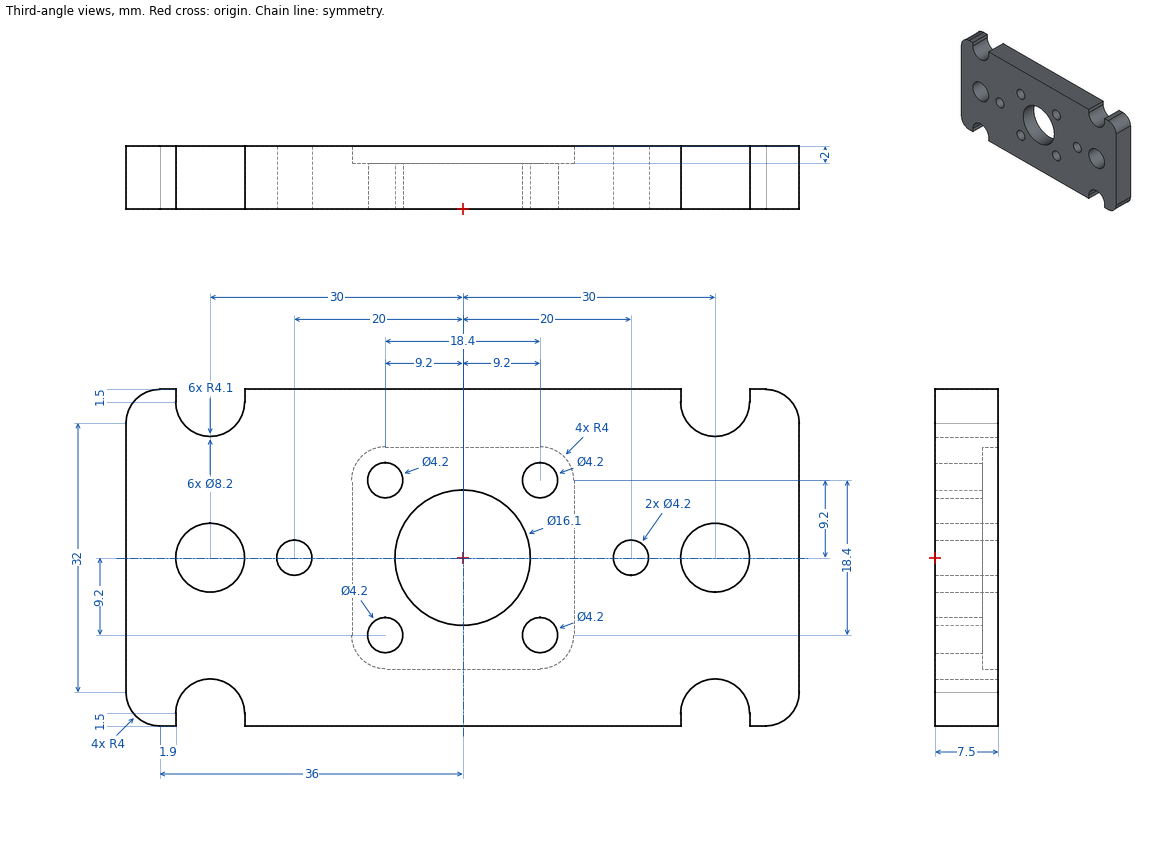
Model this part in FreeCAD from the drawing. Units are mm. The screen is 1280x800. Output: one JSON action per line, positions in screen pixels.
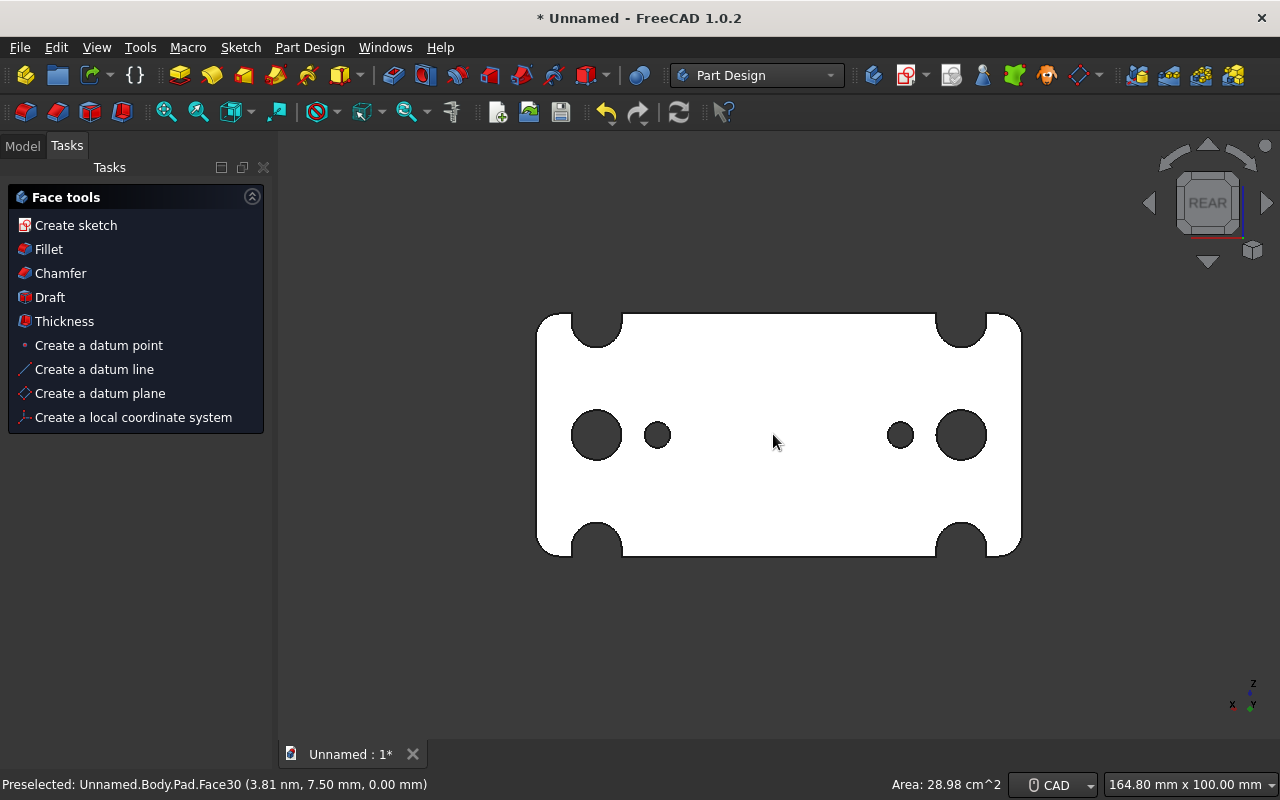
{"action": "left_click", "coordinate": [906, 76]}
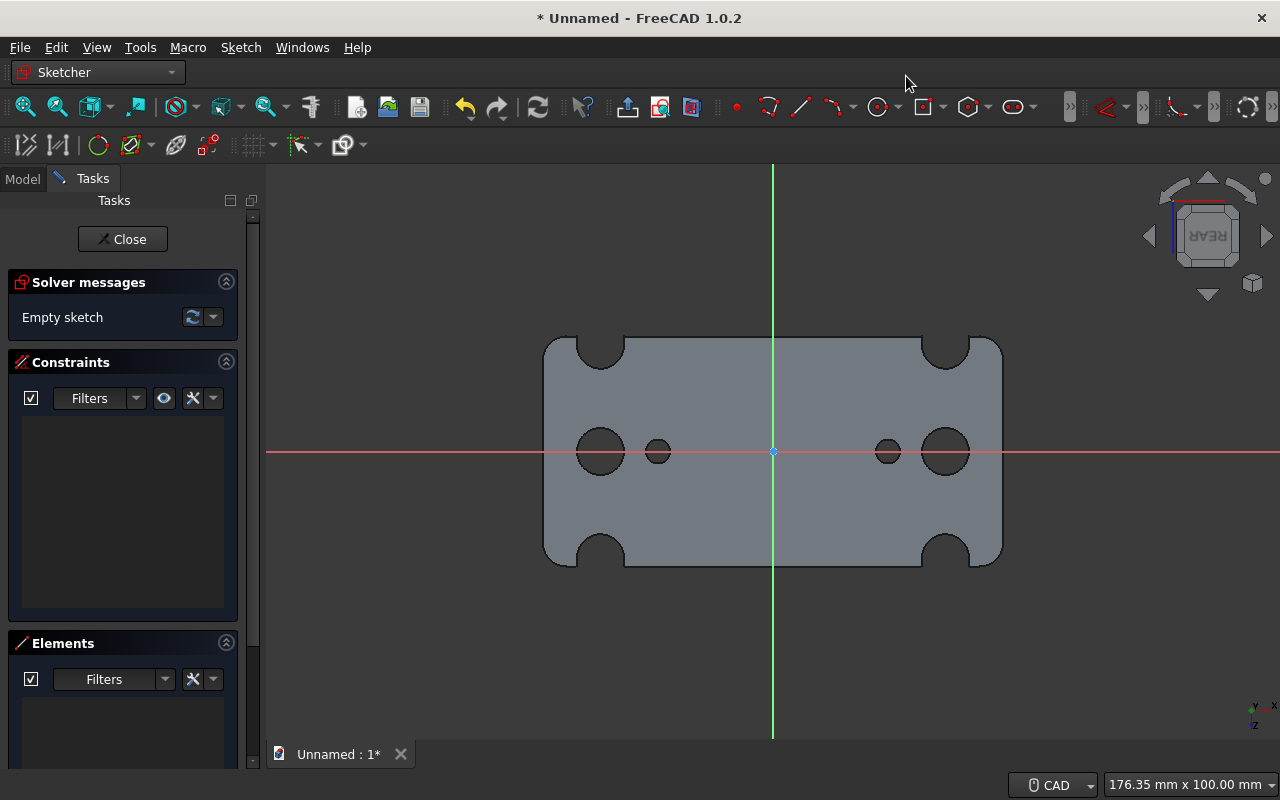
{"action": "scroll", "coordinate": [829, 452], "scroll_direction": "up", "scroll_amount": 4}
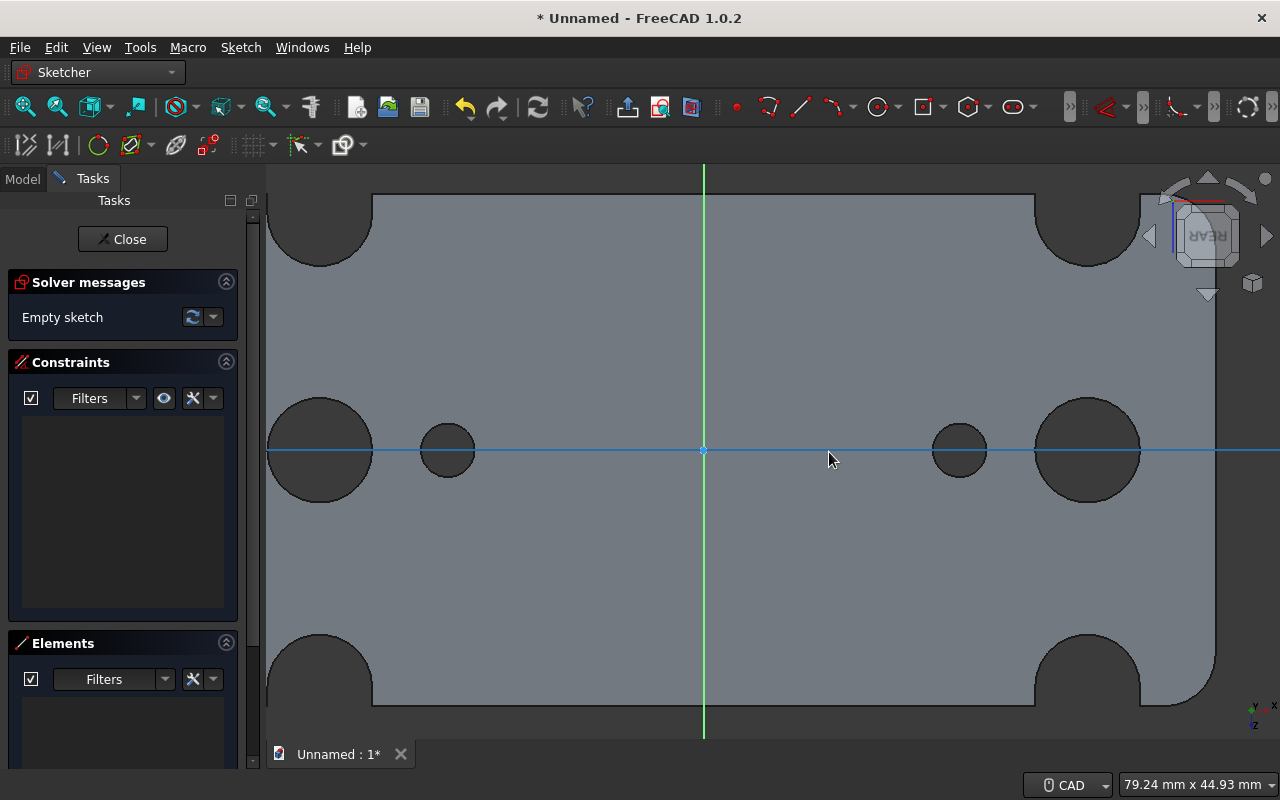
{"action": "left_click", "coordinate": [802, 108]}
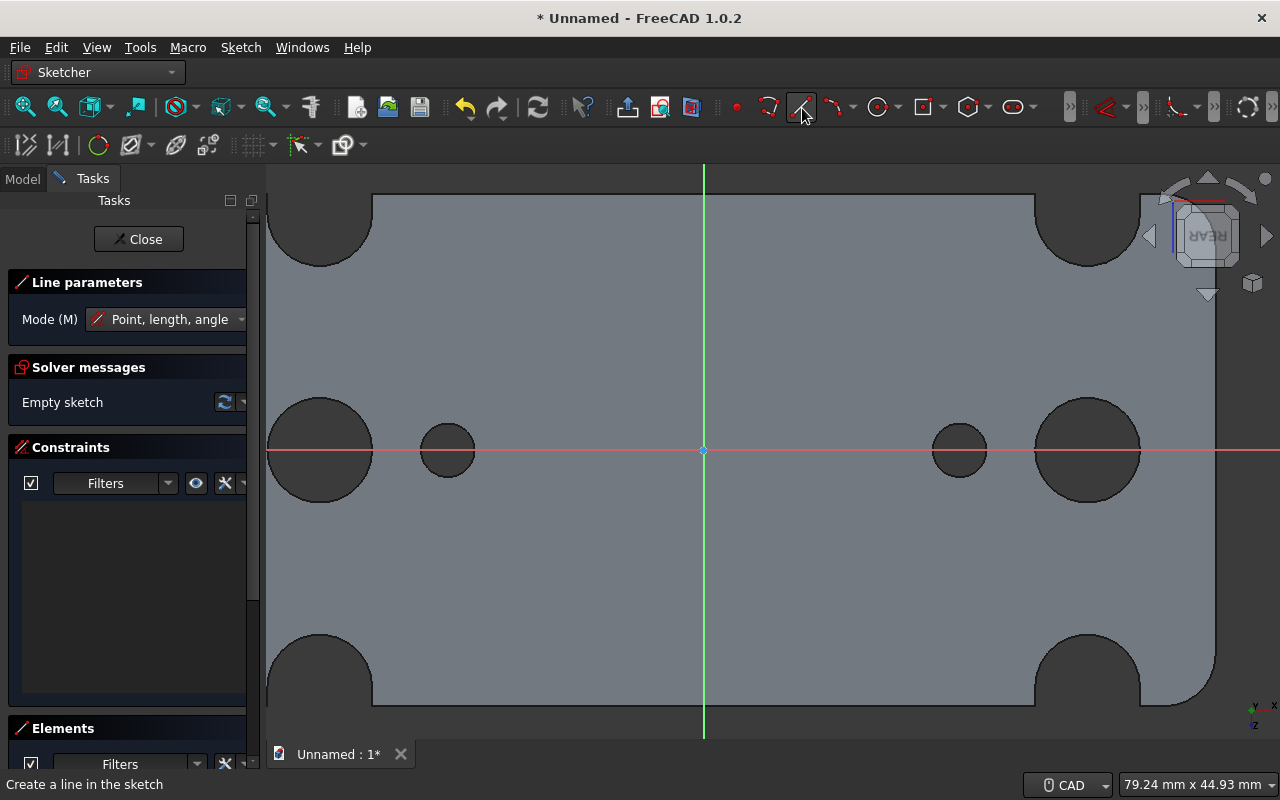
{"action": "left_click", "coordinate": [586, 619]}
{"action": "left_click", "coordinate": [821, 619]}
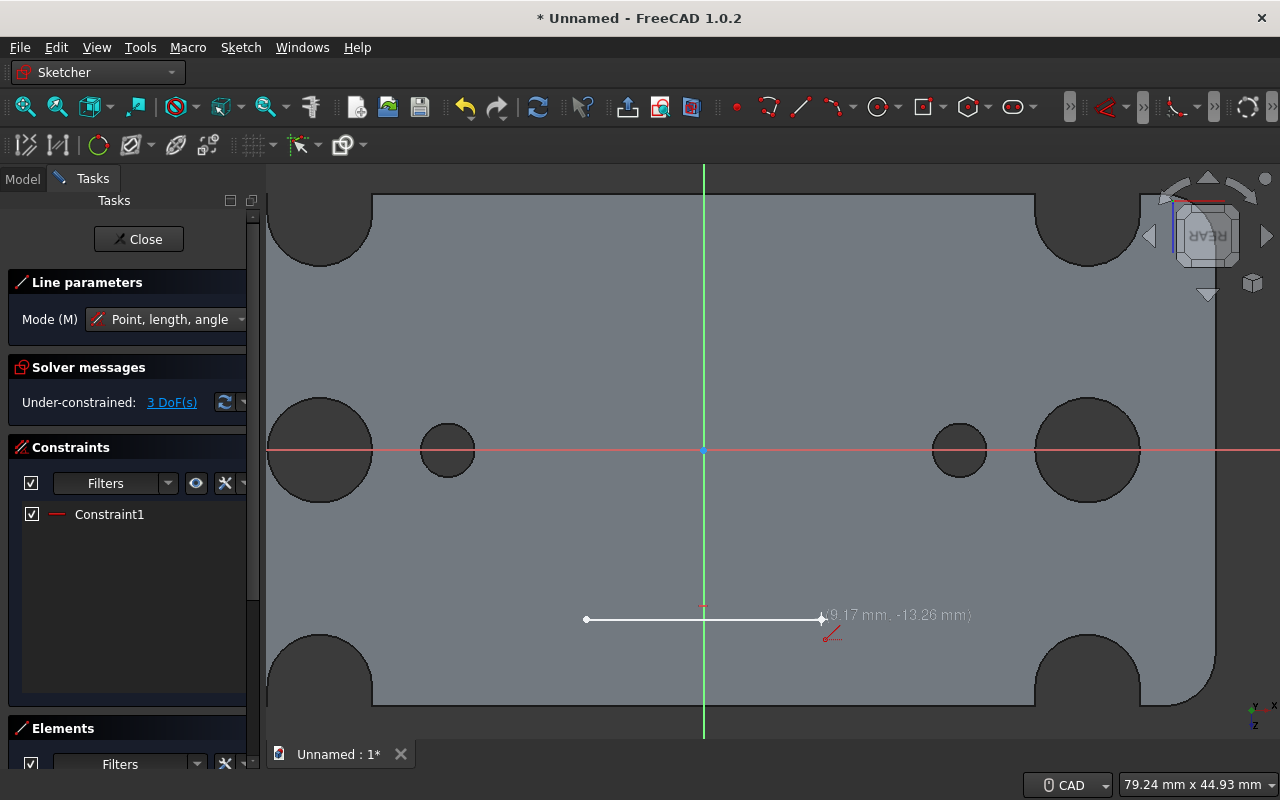
{"action": "left_click", "coordinate": [873, 568]}
{"action": "left_click", "coordinate": [873, 333]}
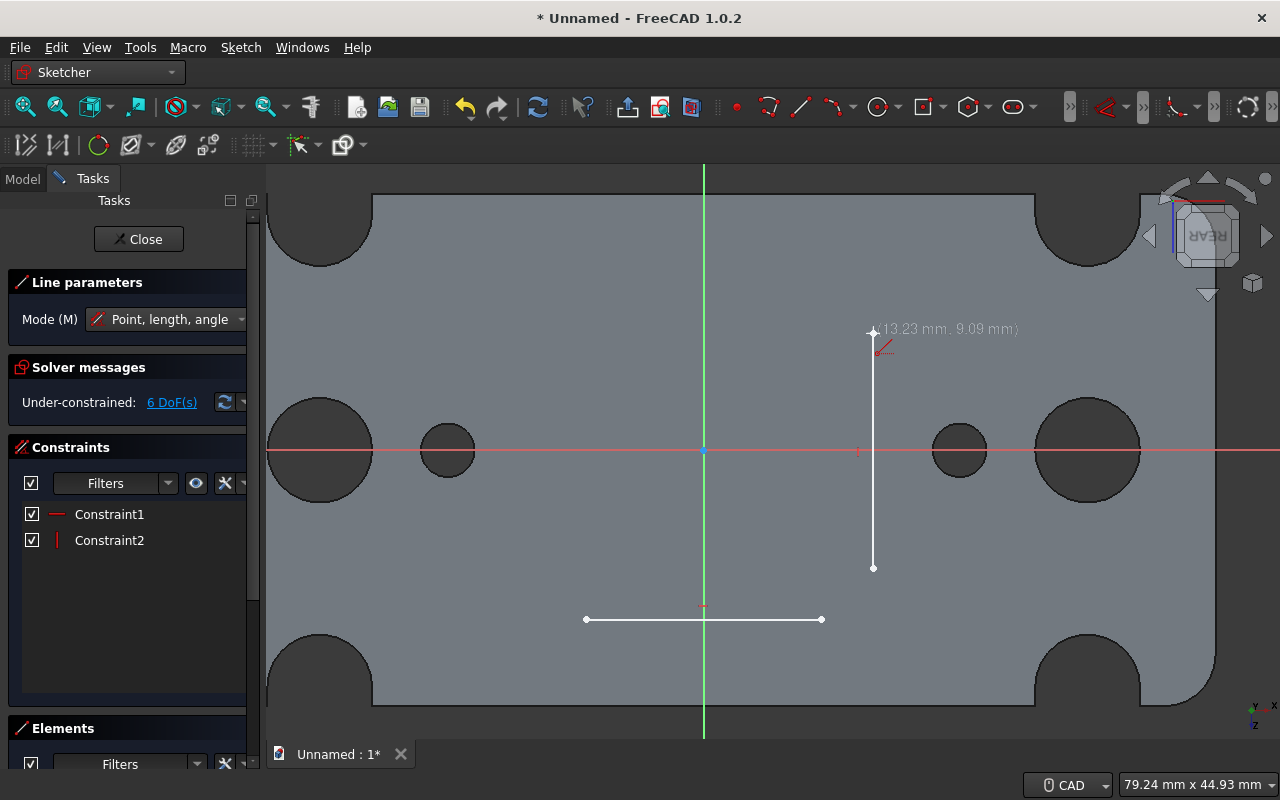
{"action": "left_click", "coordinate": [821, 281]}
{"action": "left_click", "coordinate": [586, 281]}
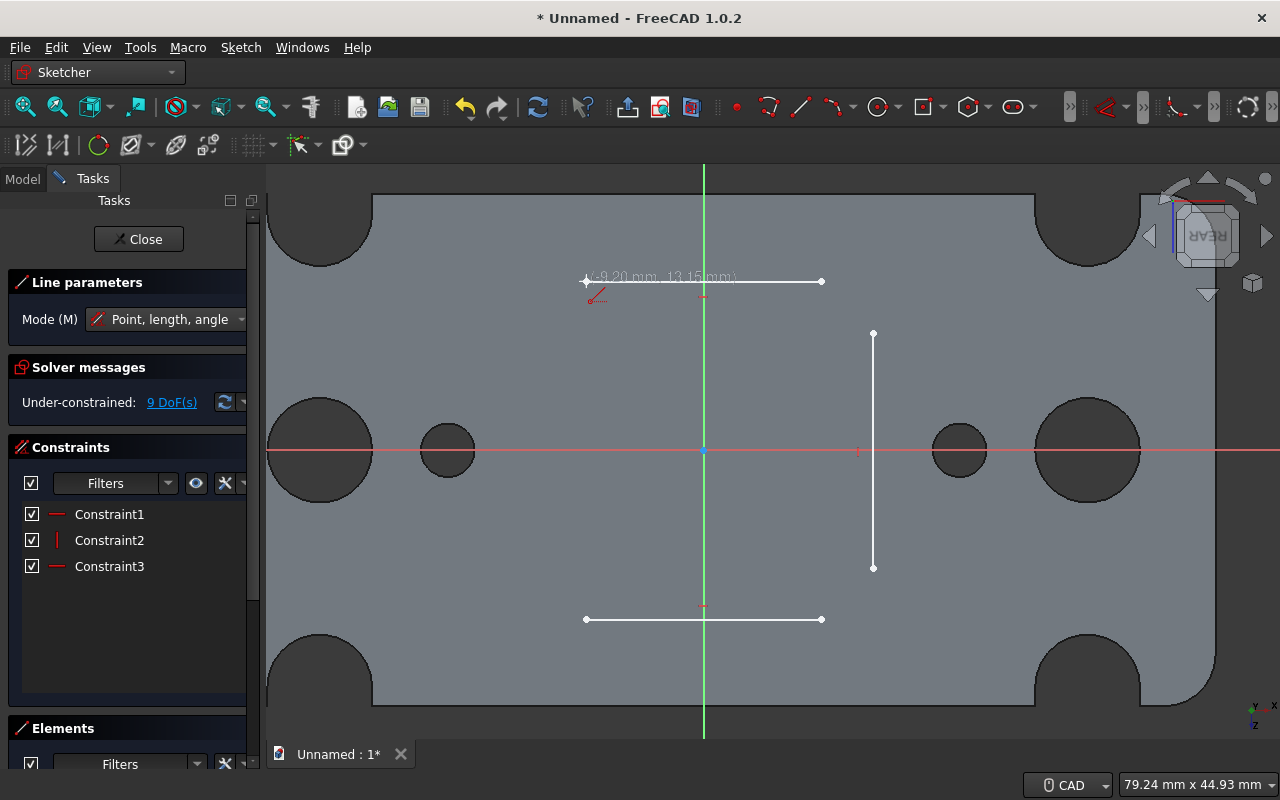
{"action": "left_click", "coordinate": [535, 333]}
{"action": "left_click", "coordinate": [535, 568]}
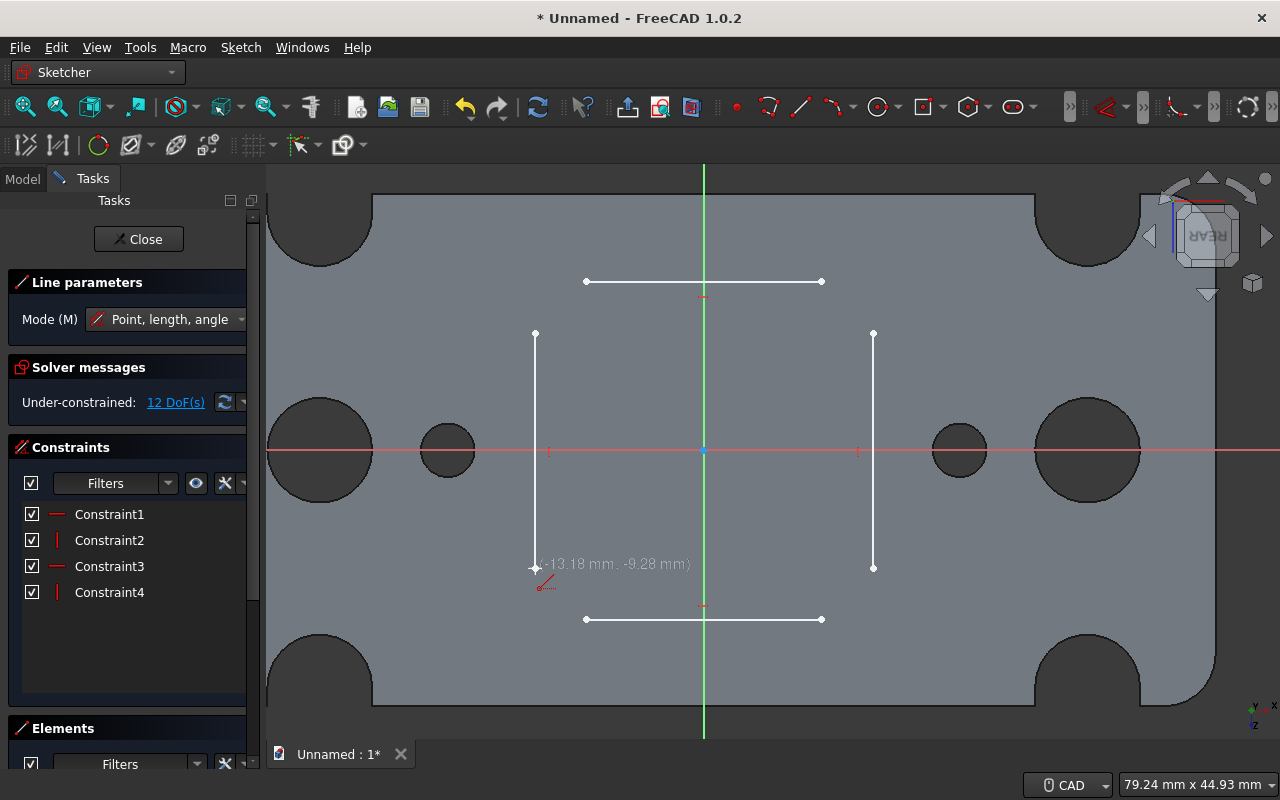
{"action": "left_click", "coordinate": [834, 108]}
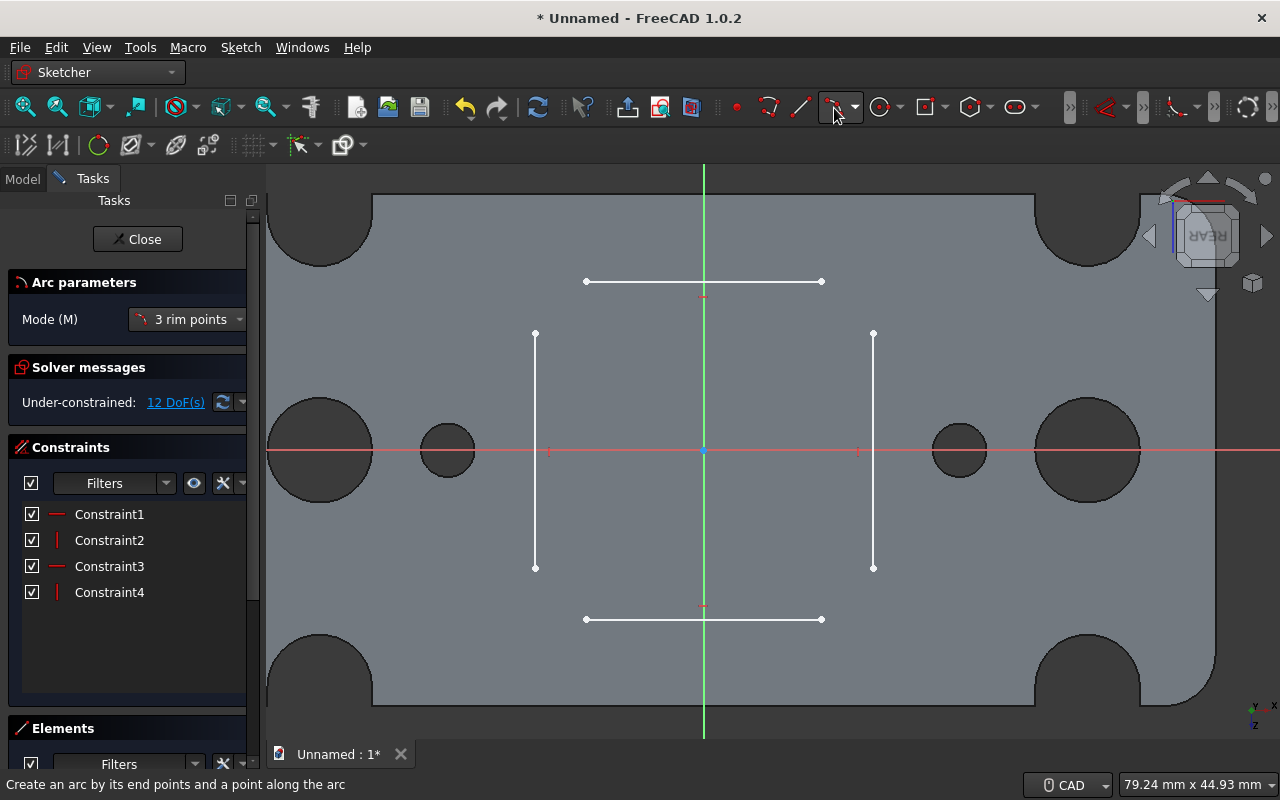
{"action": "left_click", "coordinate": [821, 620]}
{"action": "left_click", "coordinate": [873, 569]}
{"action": "left_click", "coordinate": [858, 604]}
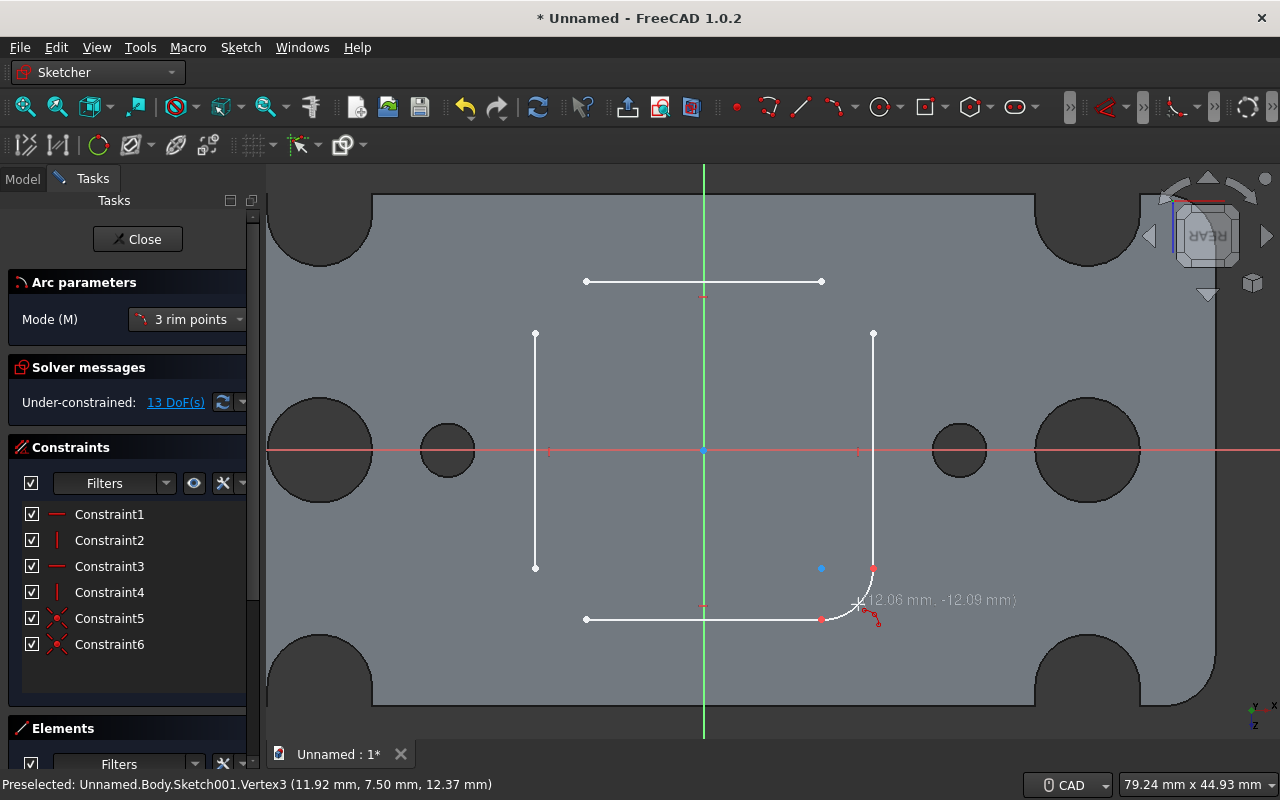
{"action": "left_click", "coordinate": [873, 334]}
{"action": "left_click", "coordinate": [821, 282]}
{"action": "left_click", "coordinate": [858, 296]}